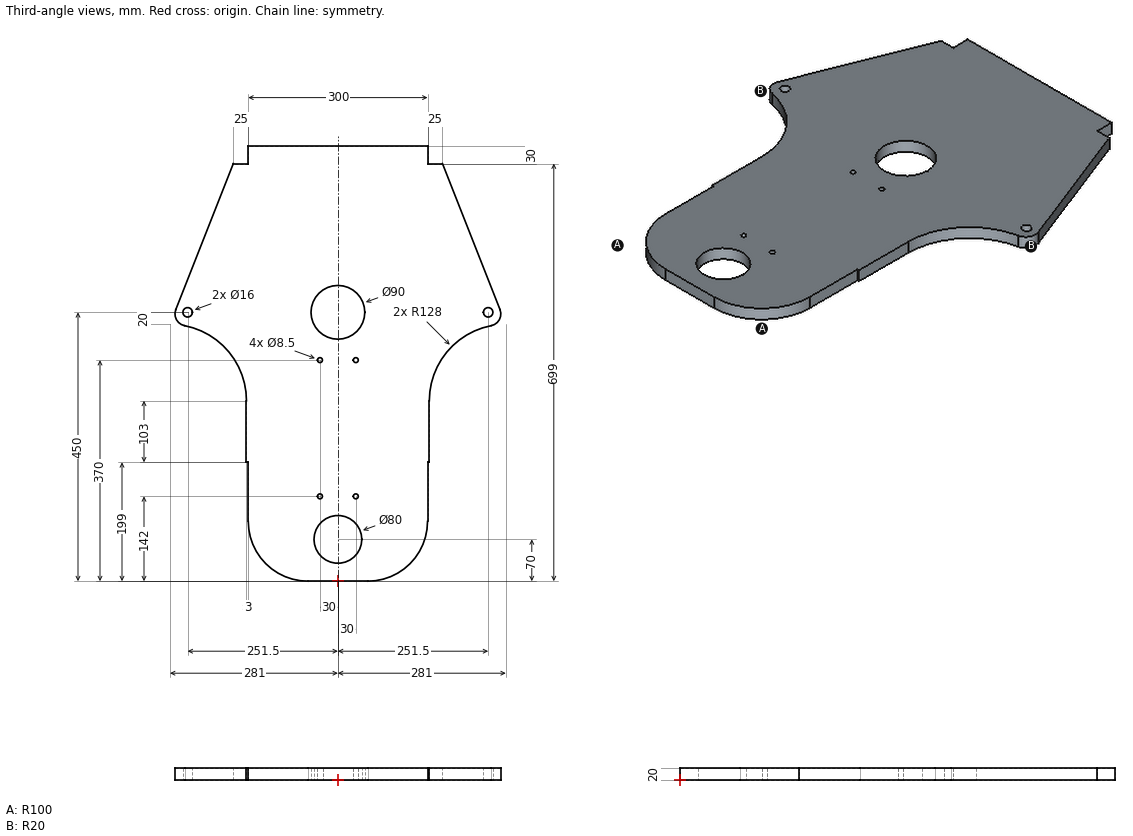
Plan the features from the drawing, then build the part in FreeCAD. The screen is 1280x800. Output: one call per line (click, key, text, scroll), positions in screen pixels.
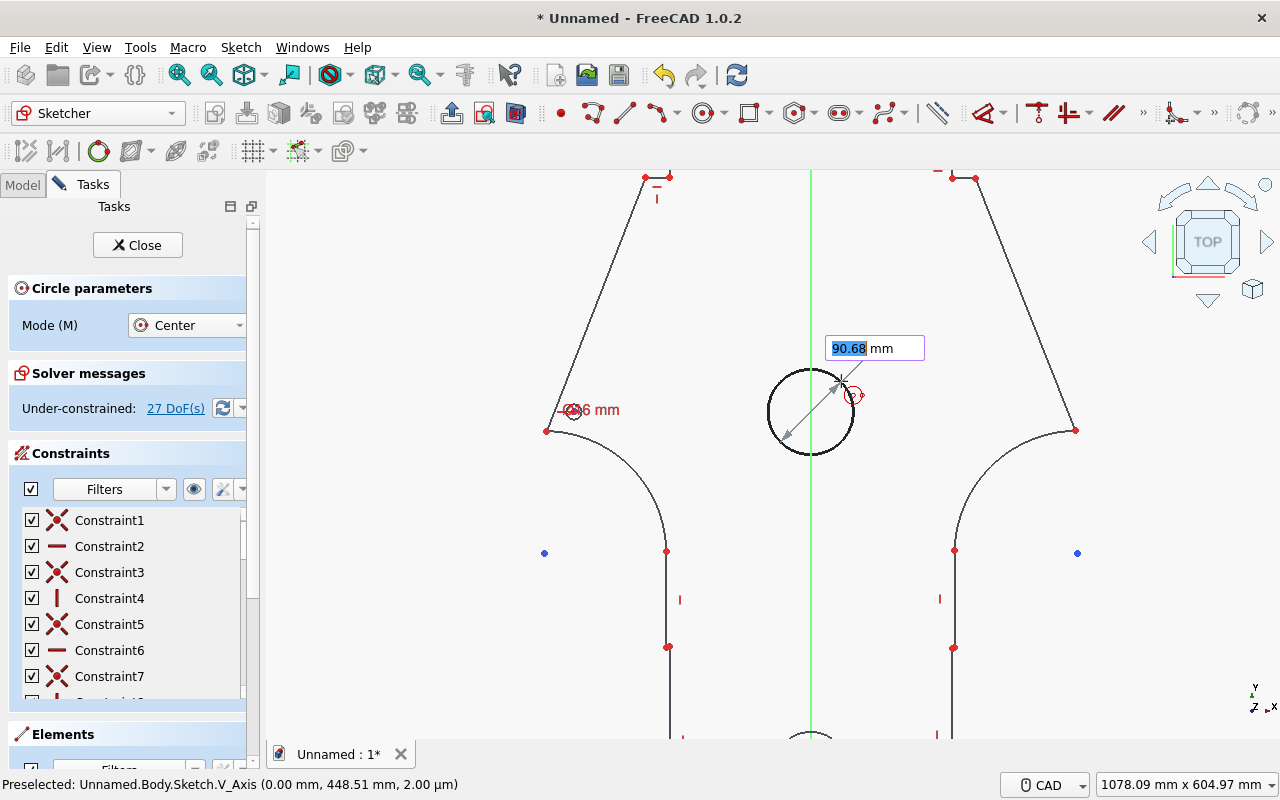
text(90)
key(Return)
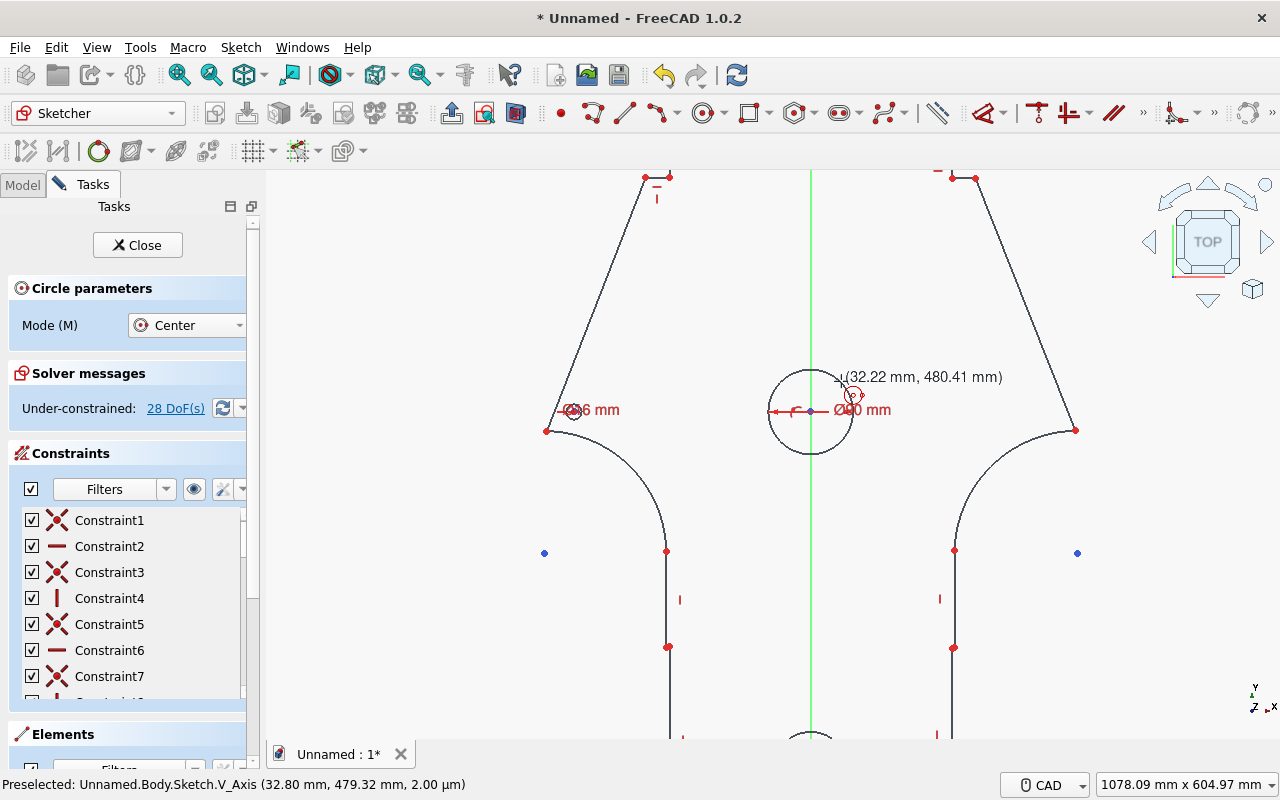
scroll(1047, 411, up, 6)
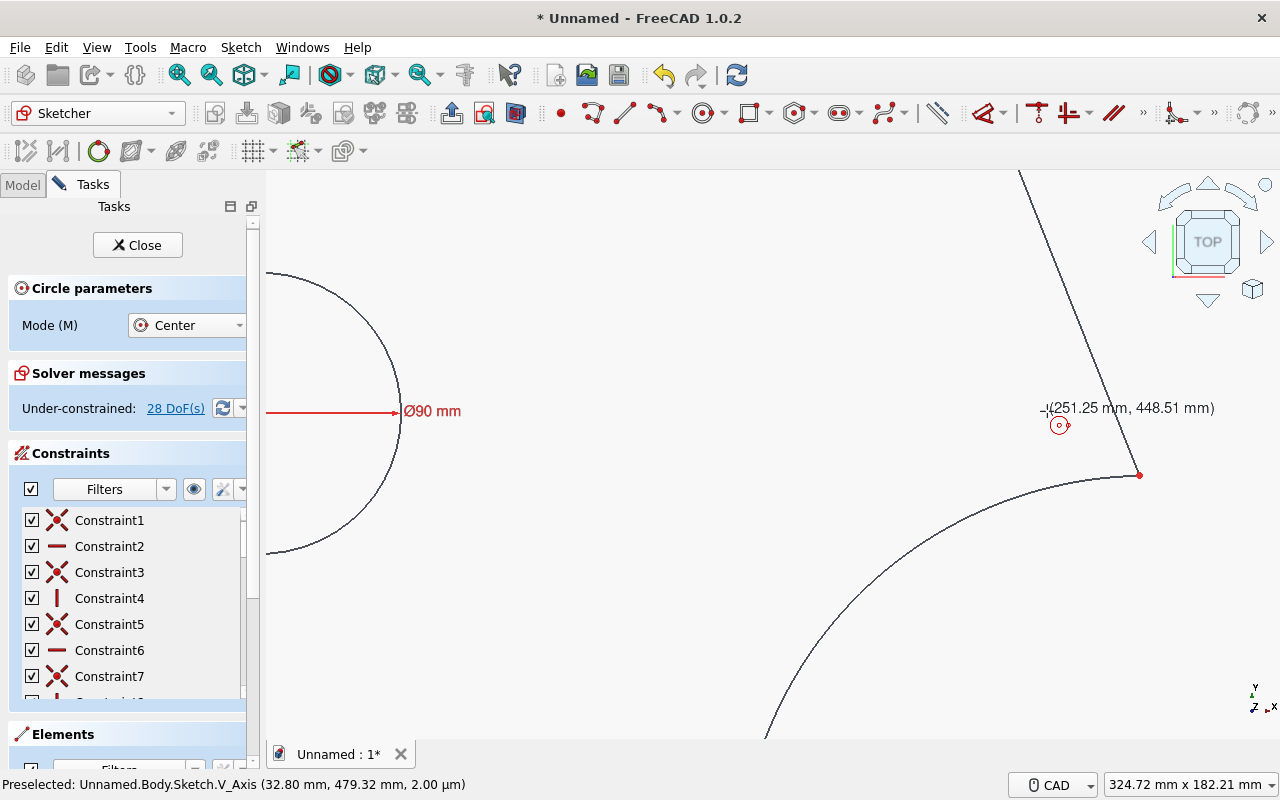
scroll(792, 411, down, 9)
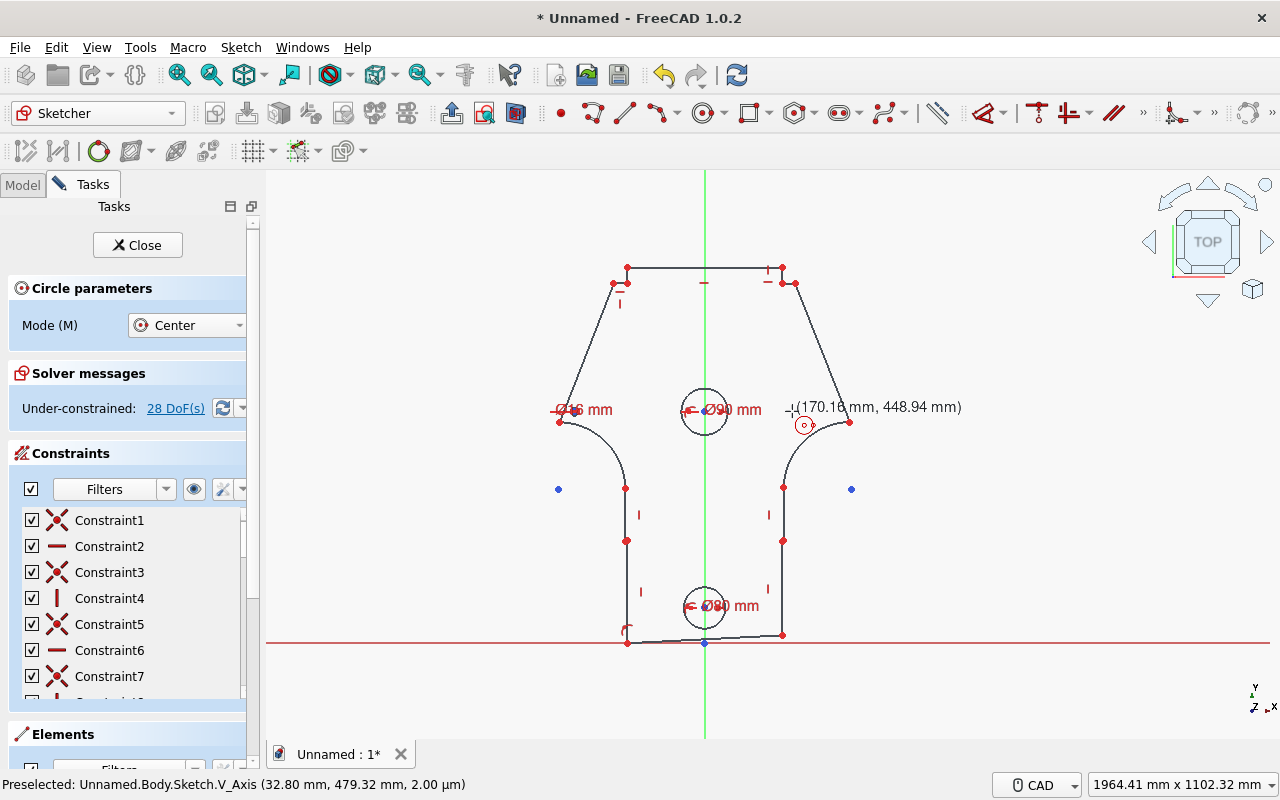
scroll(834, 411, up, 3)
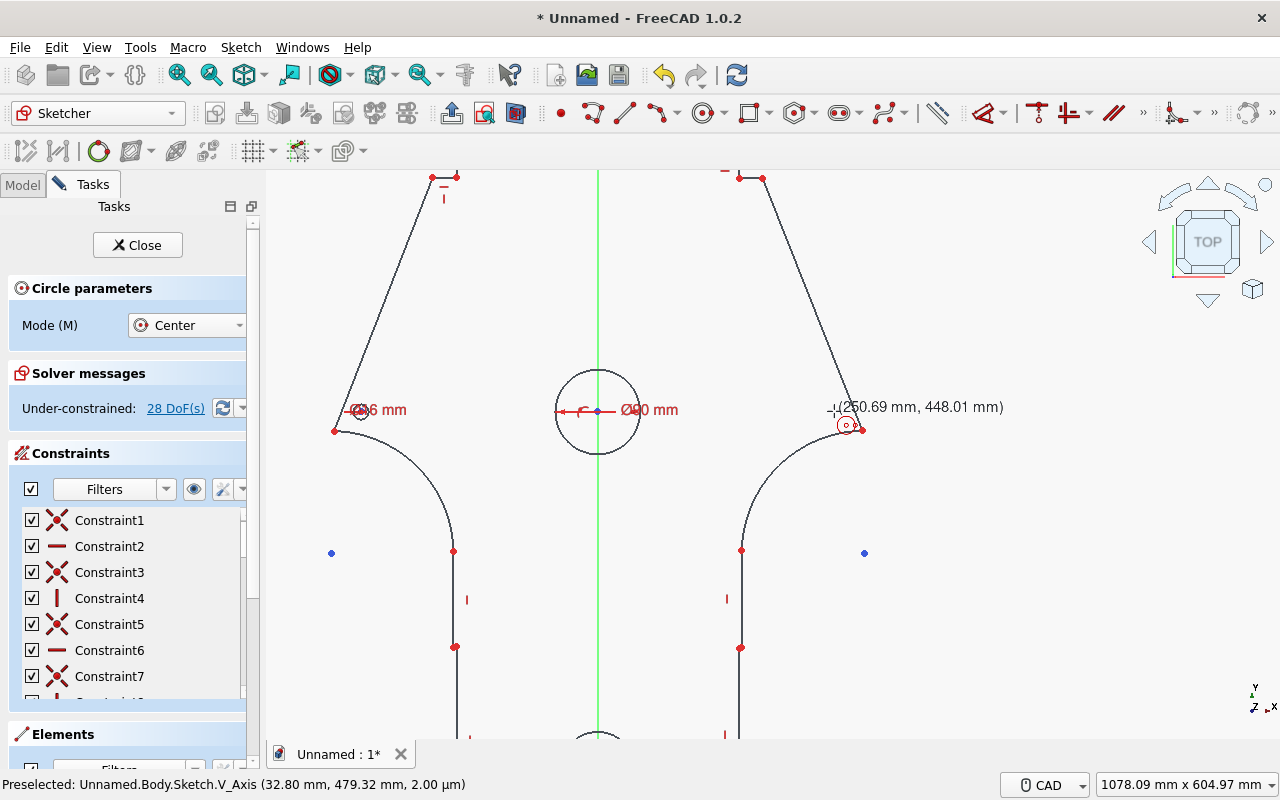
click(834, 411)
move(829, 405)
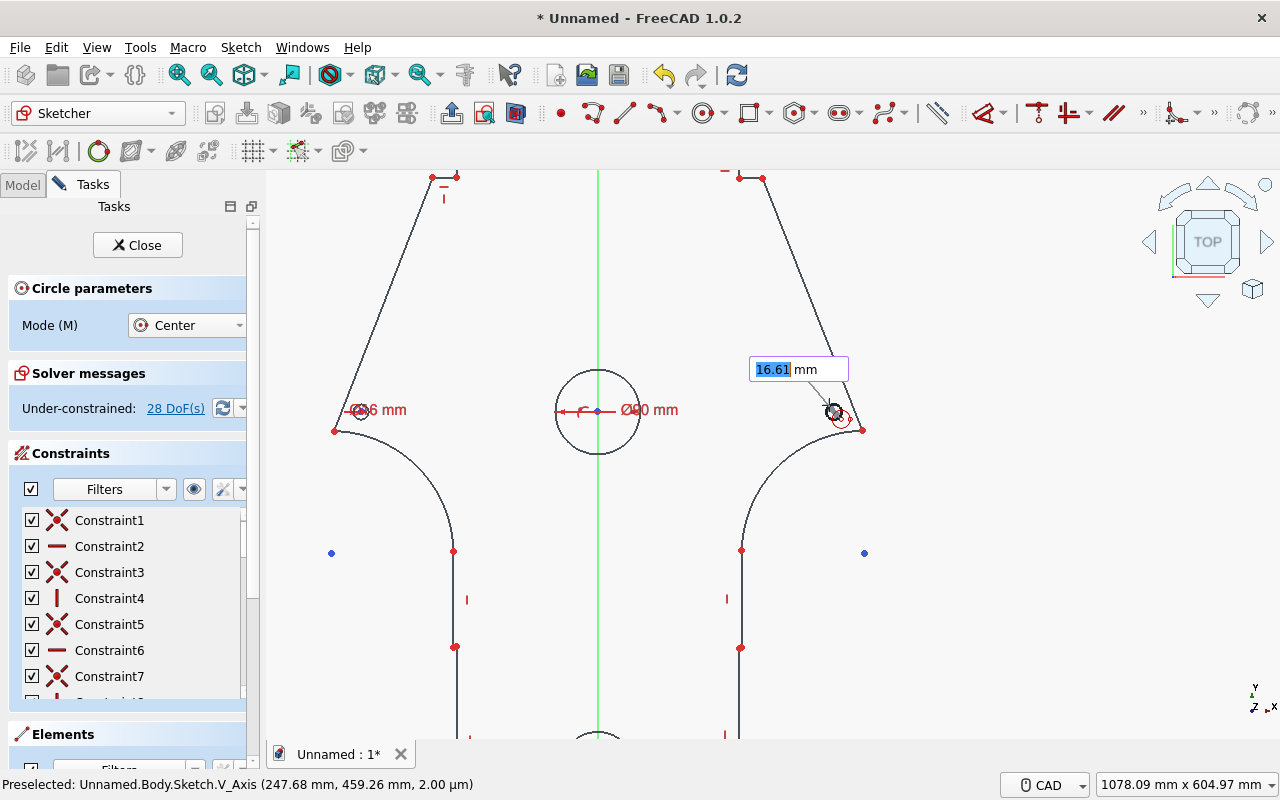
text(16)
key(Return)
key(Escape)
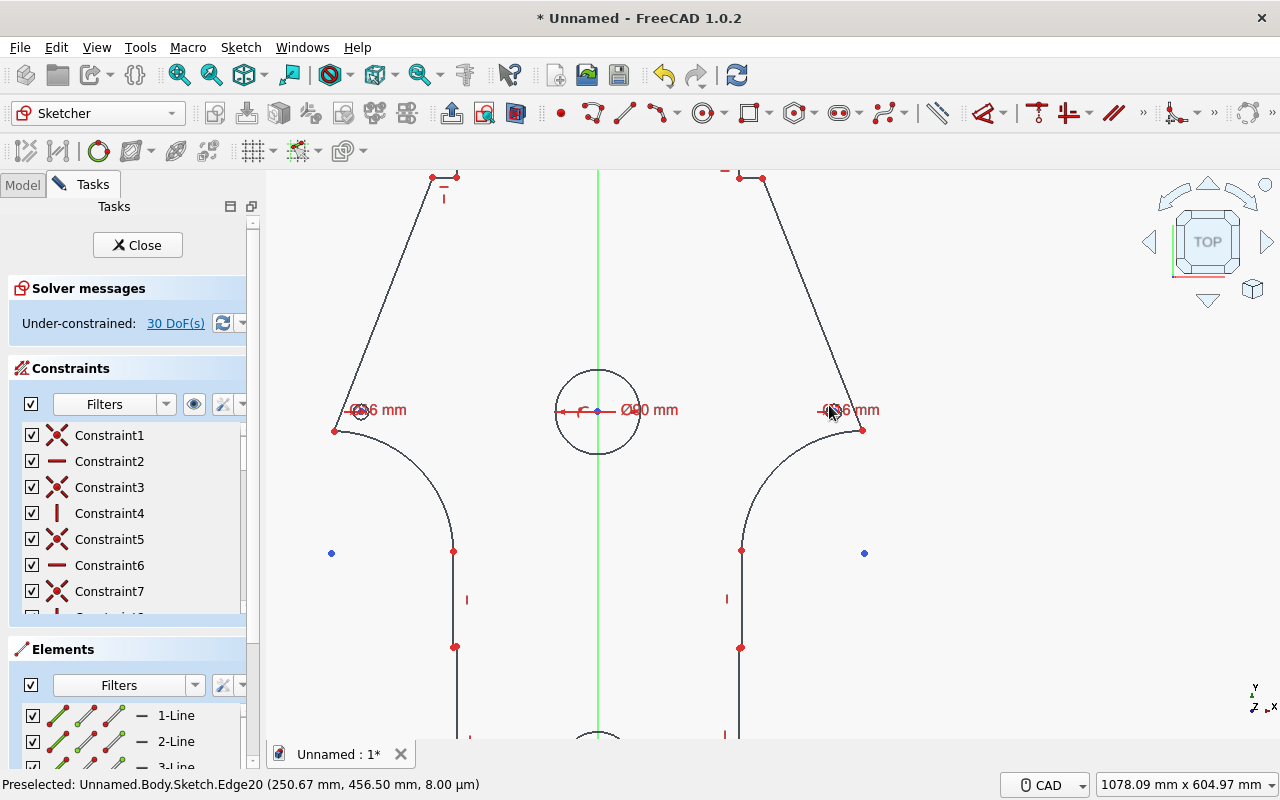
scroll(455, 647, up, 11)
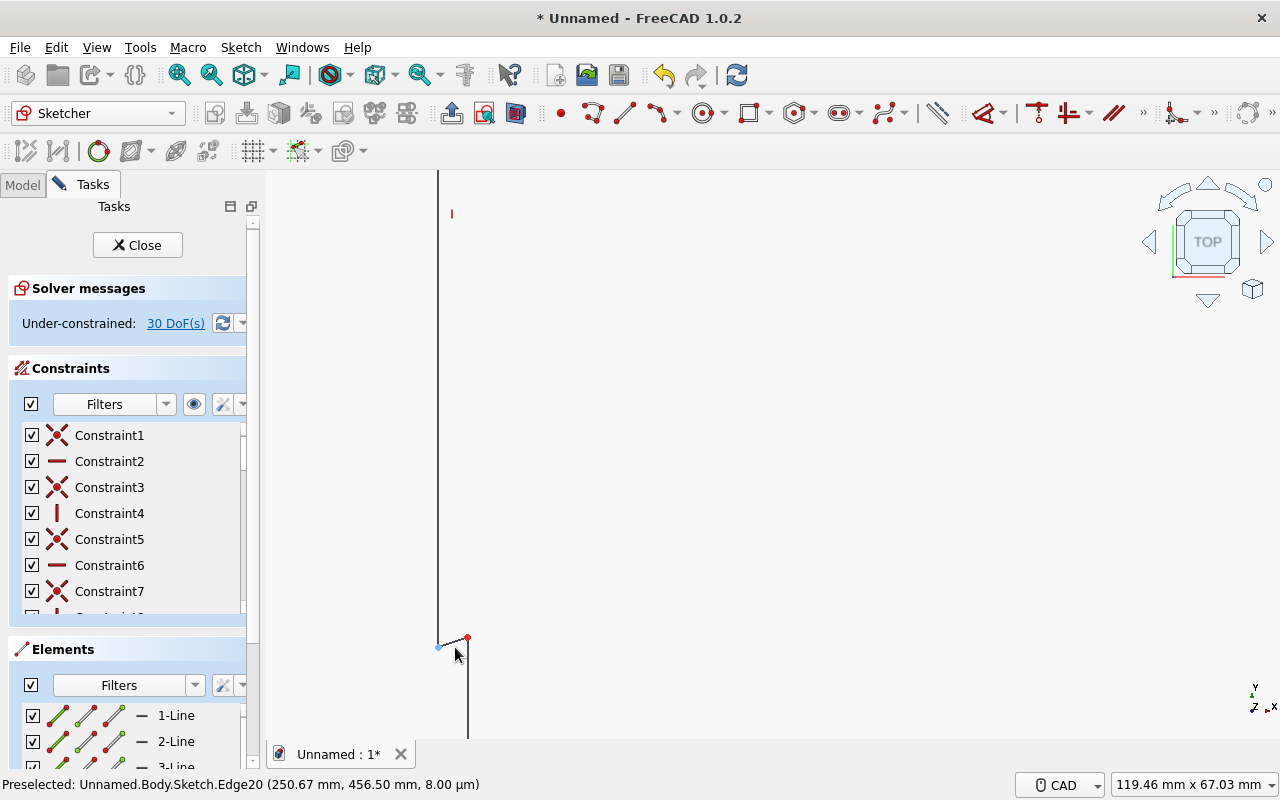
click(453, 642)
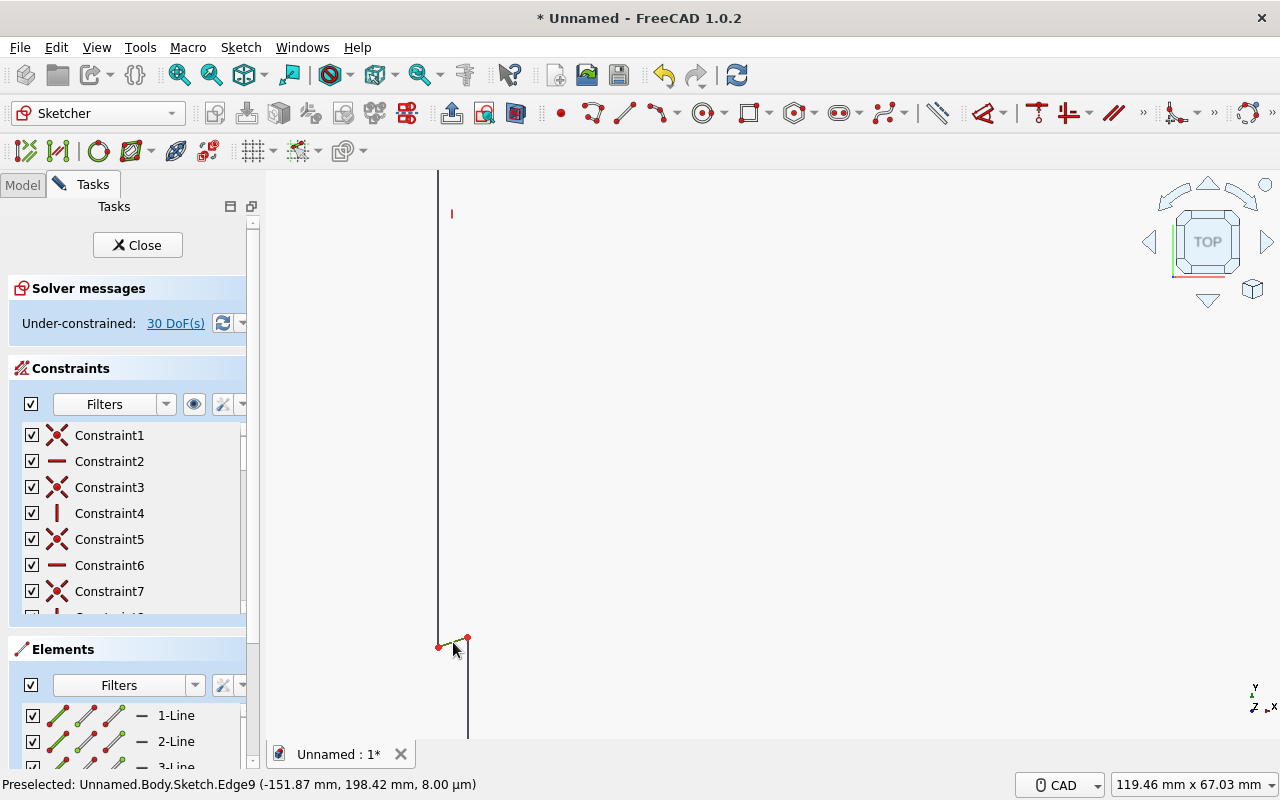
click(1092, 114)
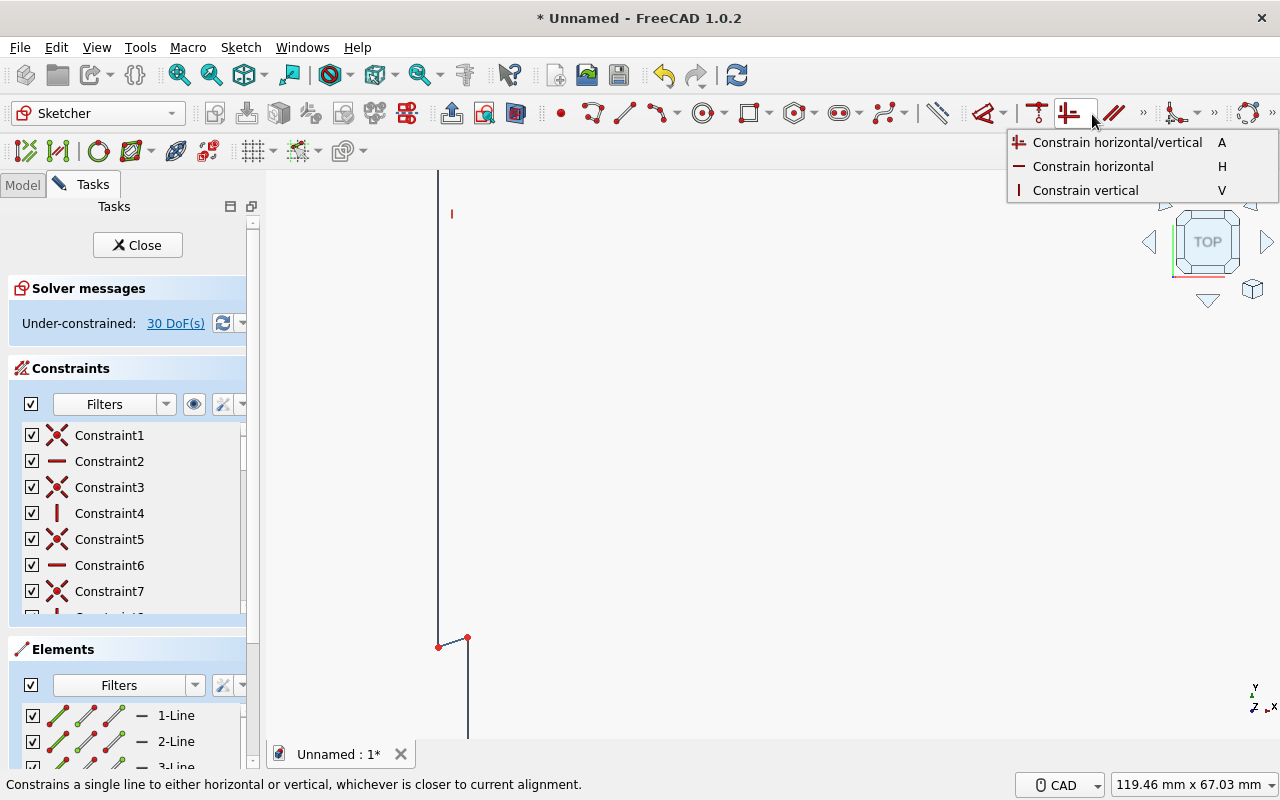
click(1143, 166)